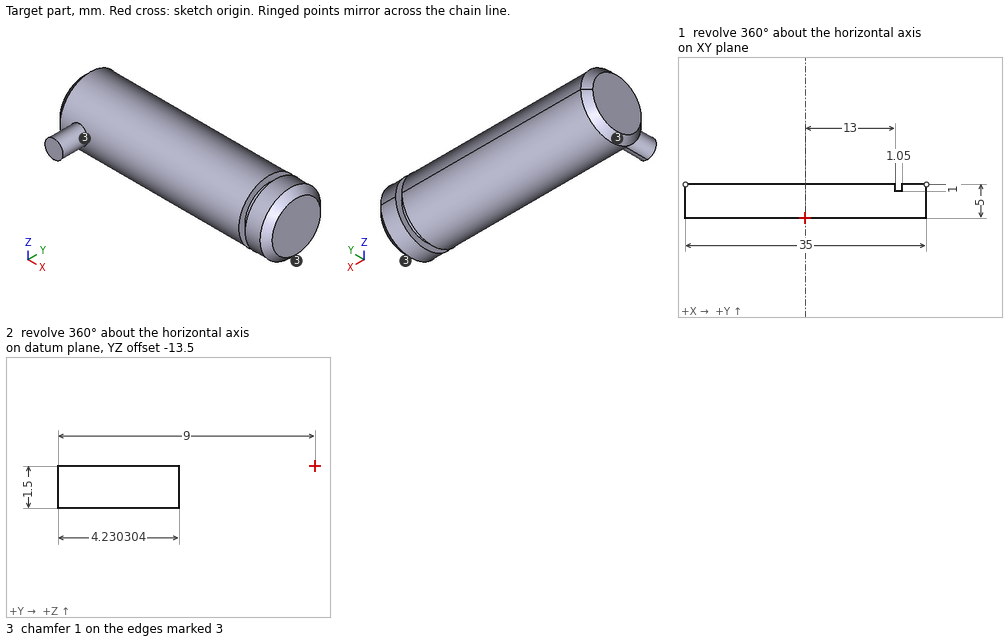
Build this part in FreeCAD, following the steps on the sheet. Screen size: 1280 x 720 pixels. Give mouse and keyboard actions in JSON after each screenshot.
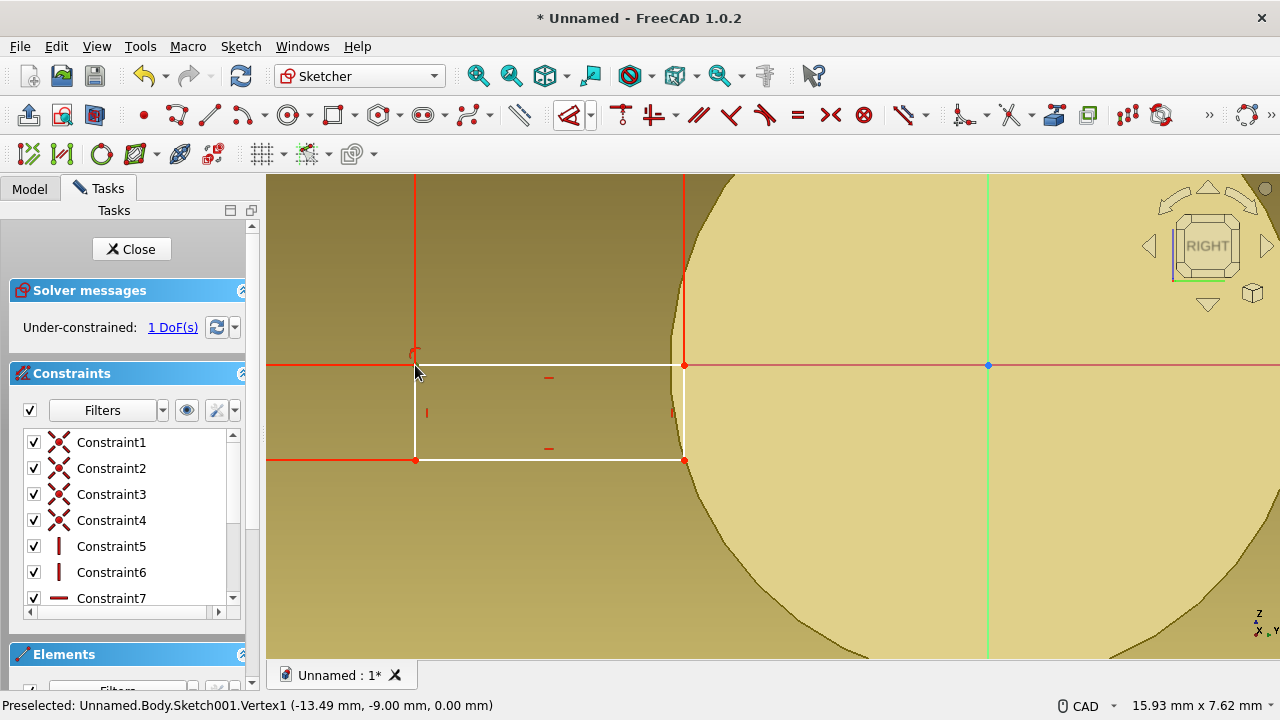
{"action": "key", "text": "l"}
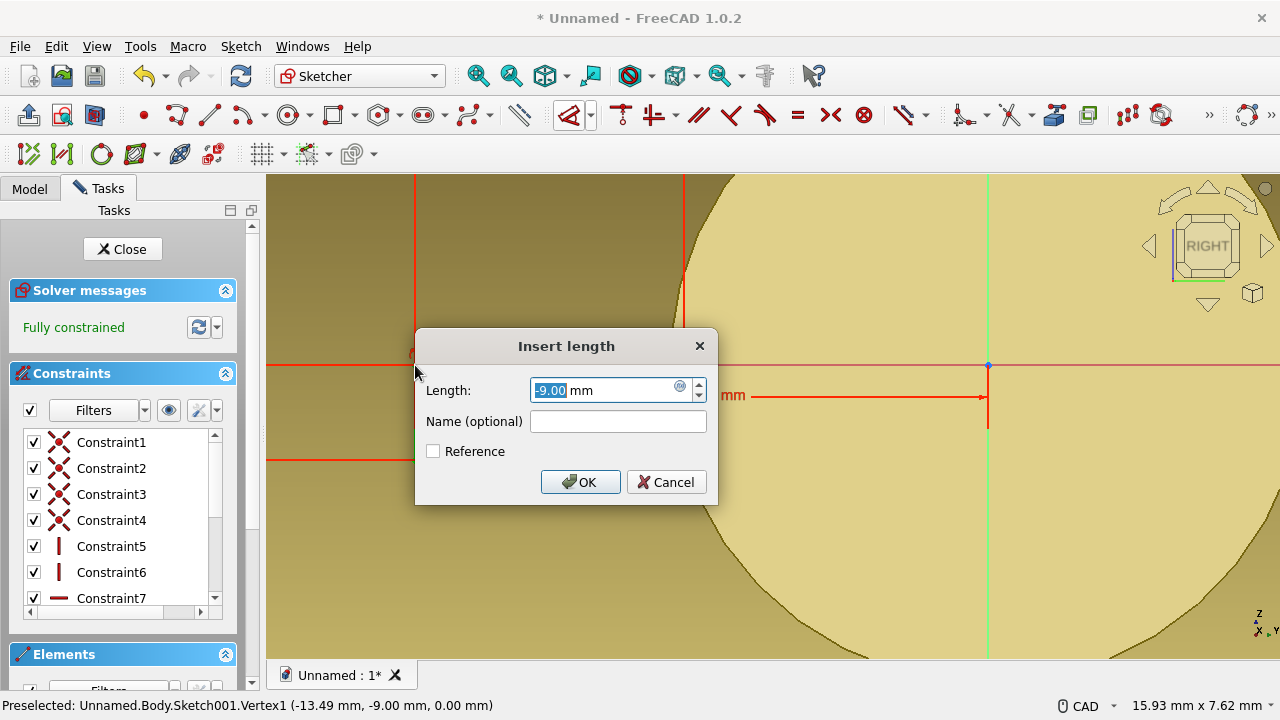
{"action": "type", "text": "-9"}
{"action": "key", "text": "Return"}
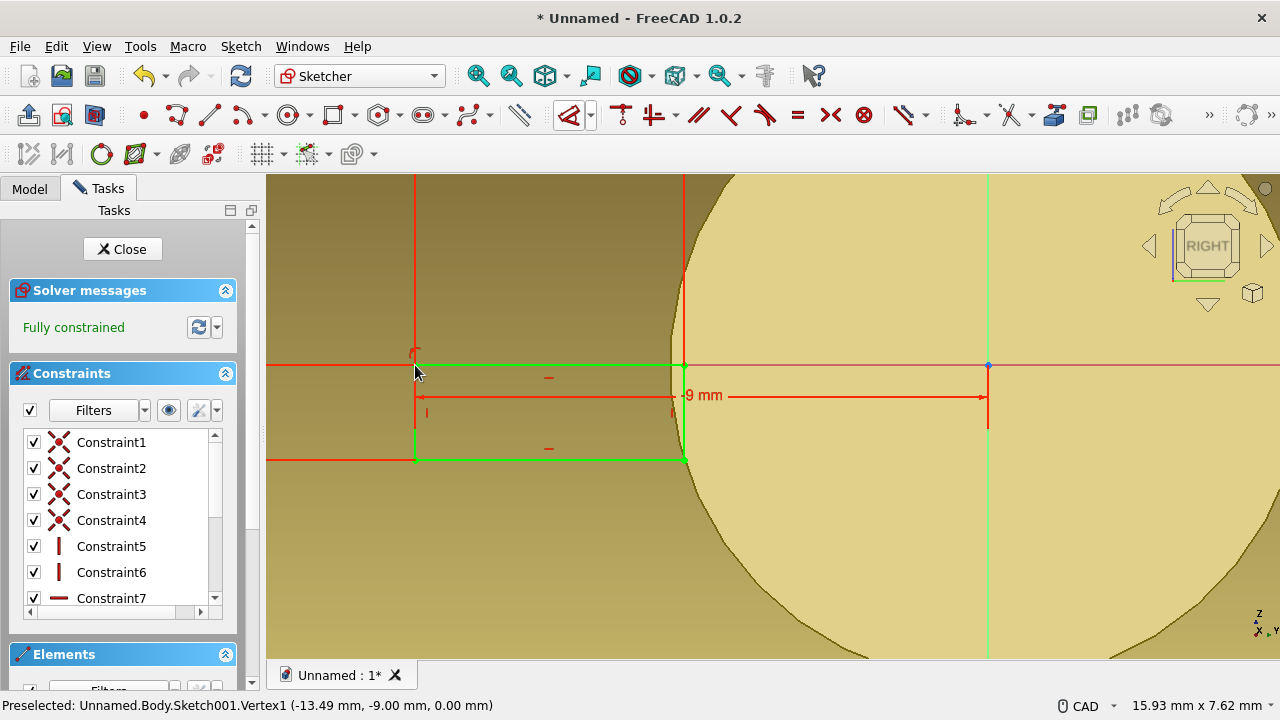
{"action": "left_click", "coordinate": [123, 249]}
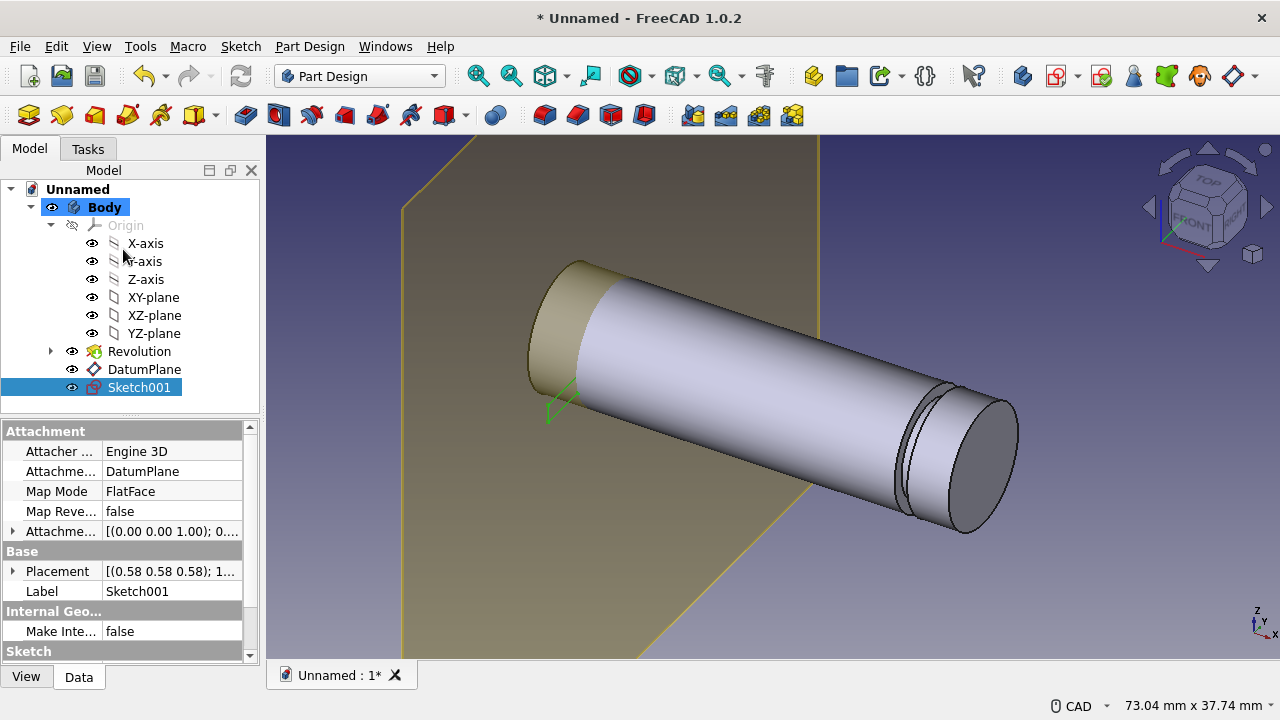
{"action": "left_click", "coordinate": [62, 116]}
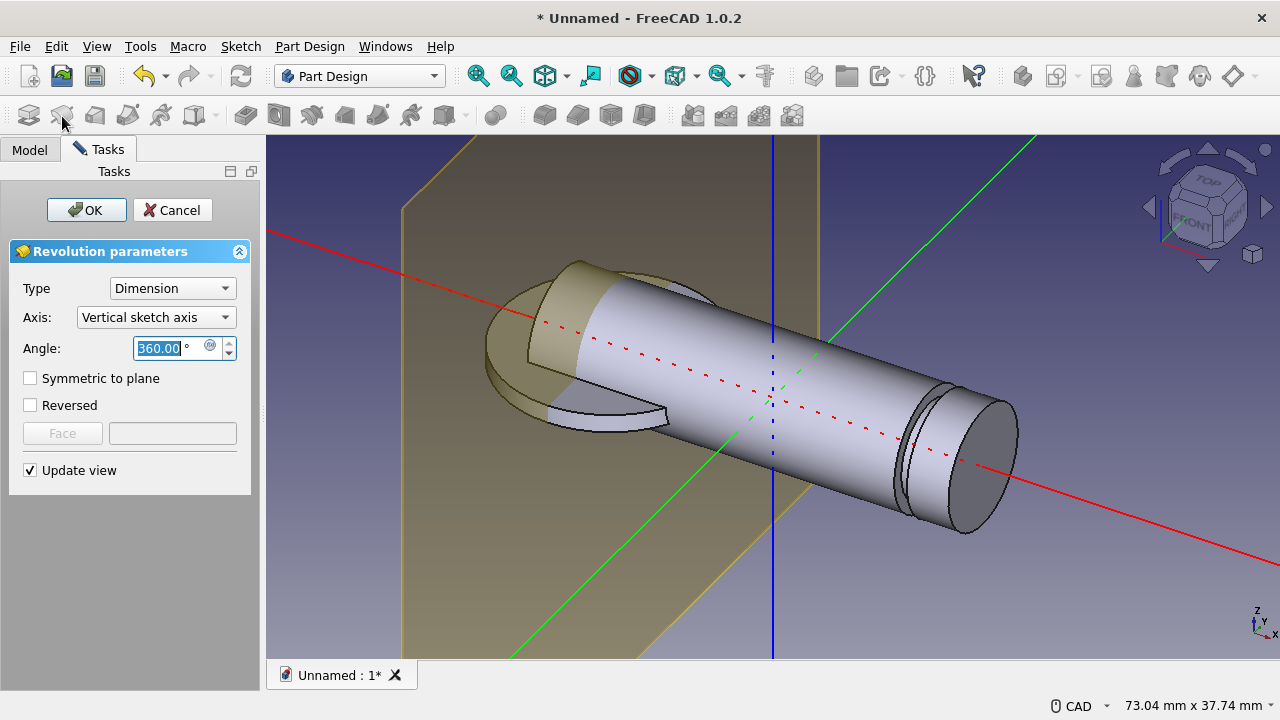
{"action": "left_click", "coordinate": [157, 318]}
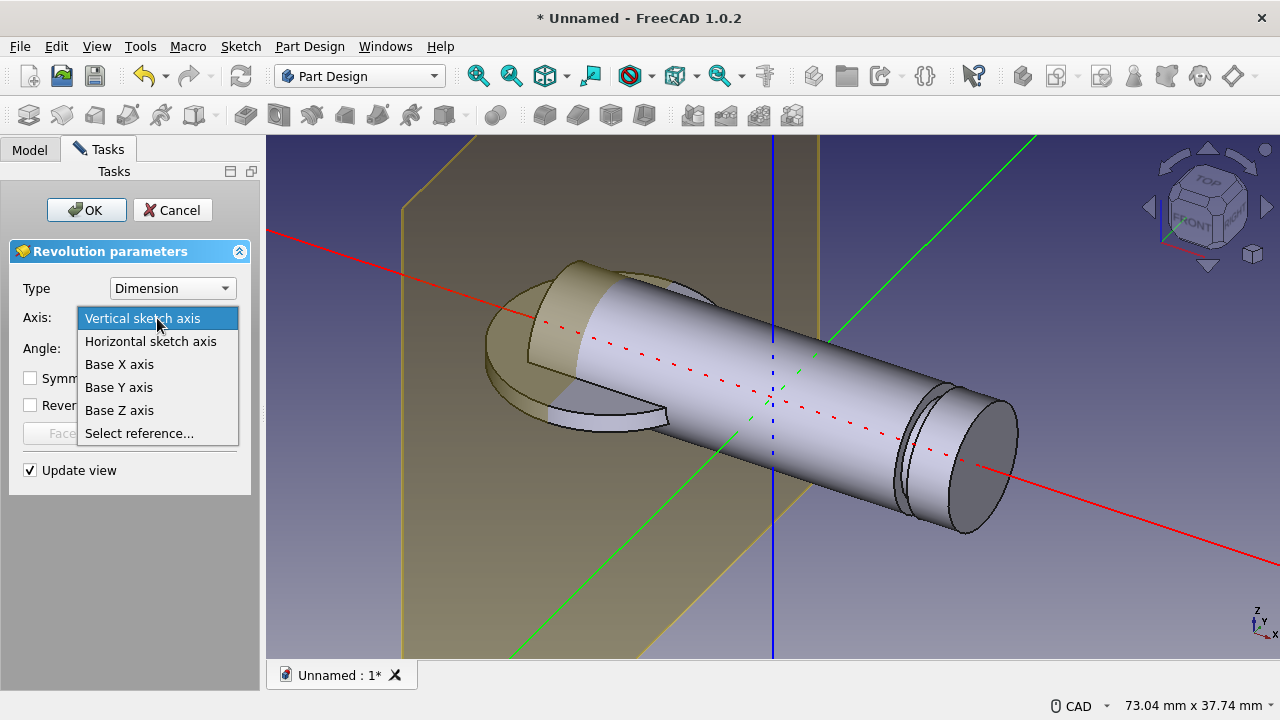
{"action": "left_click", "coordinate": [156, 342]}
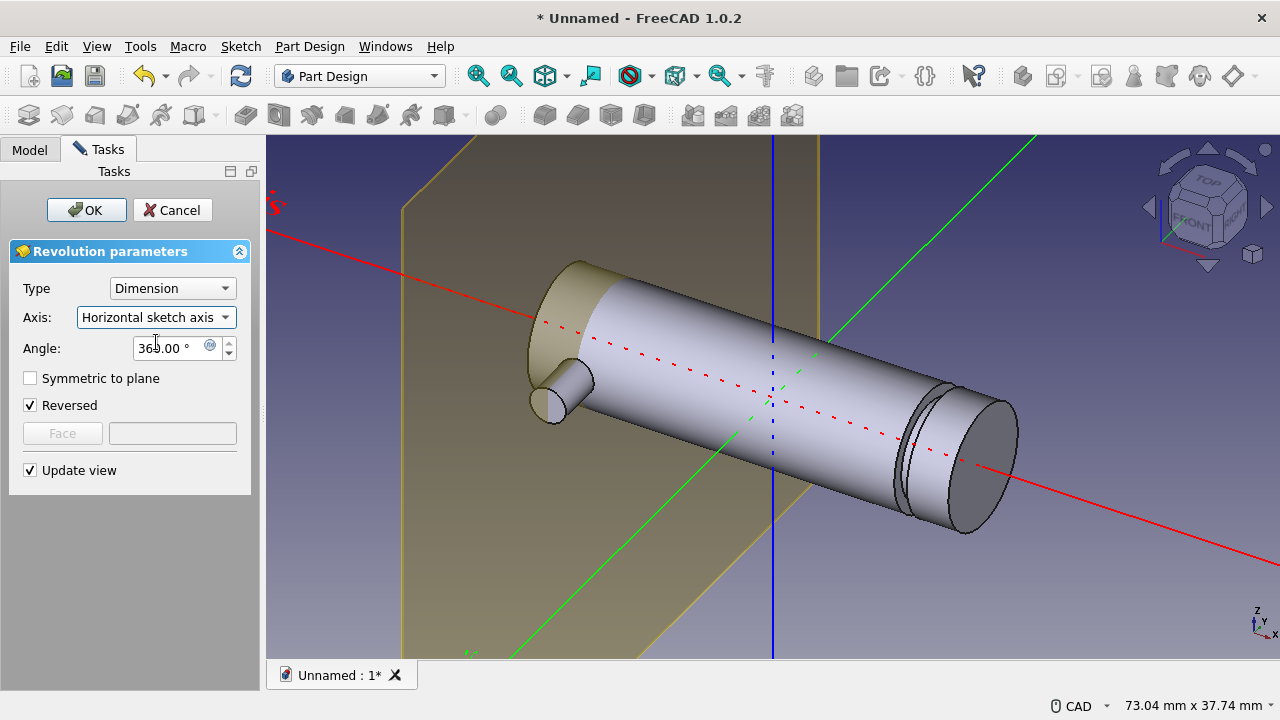
{"action": "left_click", "coordinate": [87, 210]}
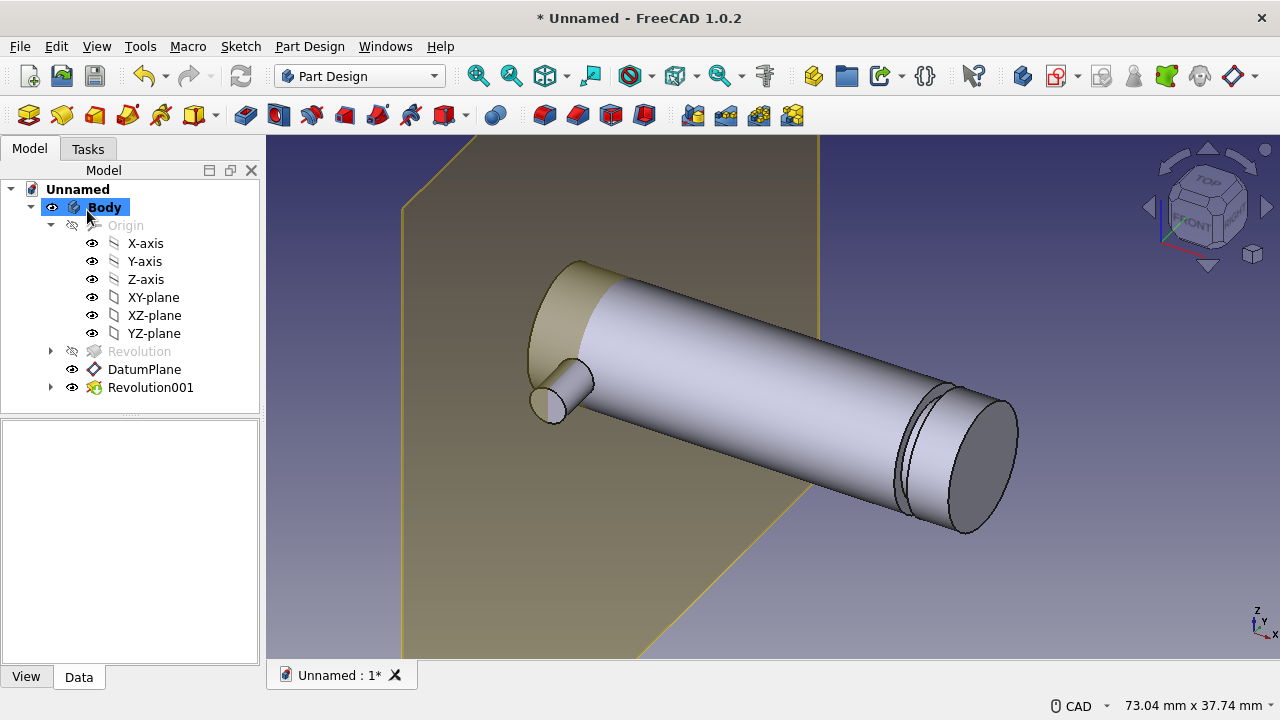
{"action": "left_click", "coordinate": [117, 369]}
{"action": "key", "text": "space"}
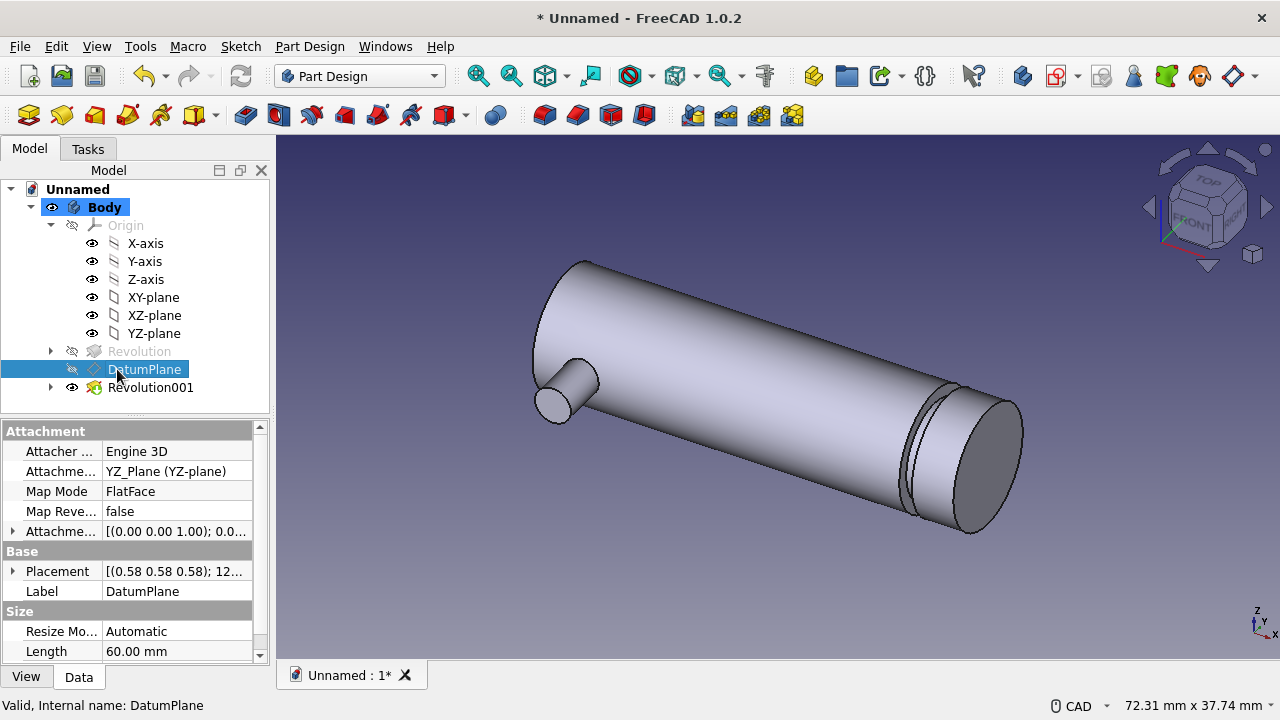
{"action": "left_click", "coordinate": [953, 500]}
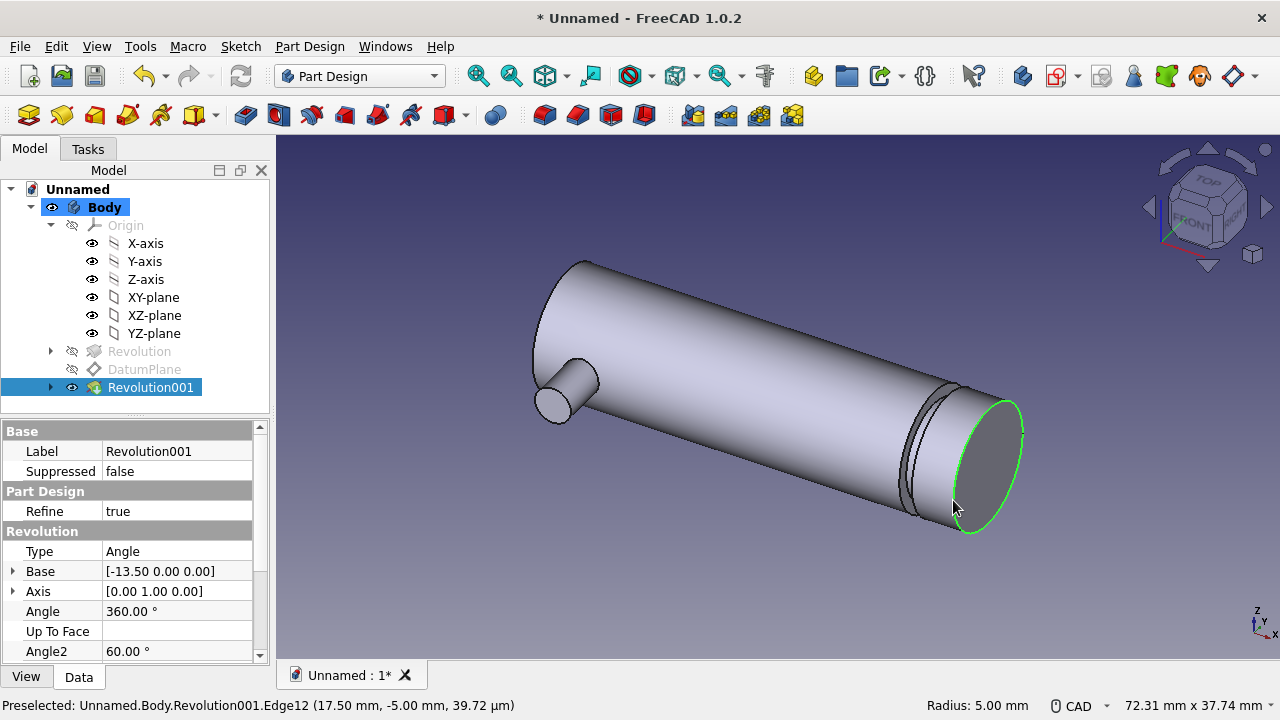
{"action": "key", "text": "0"}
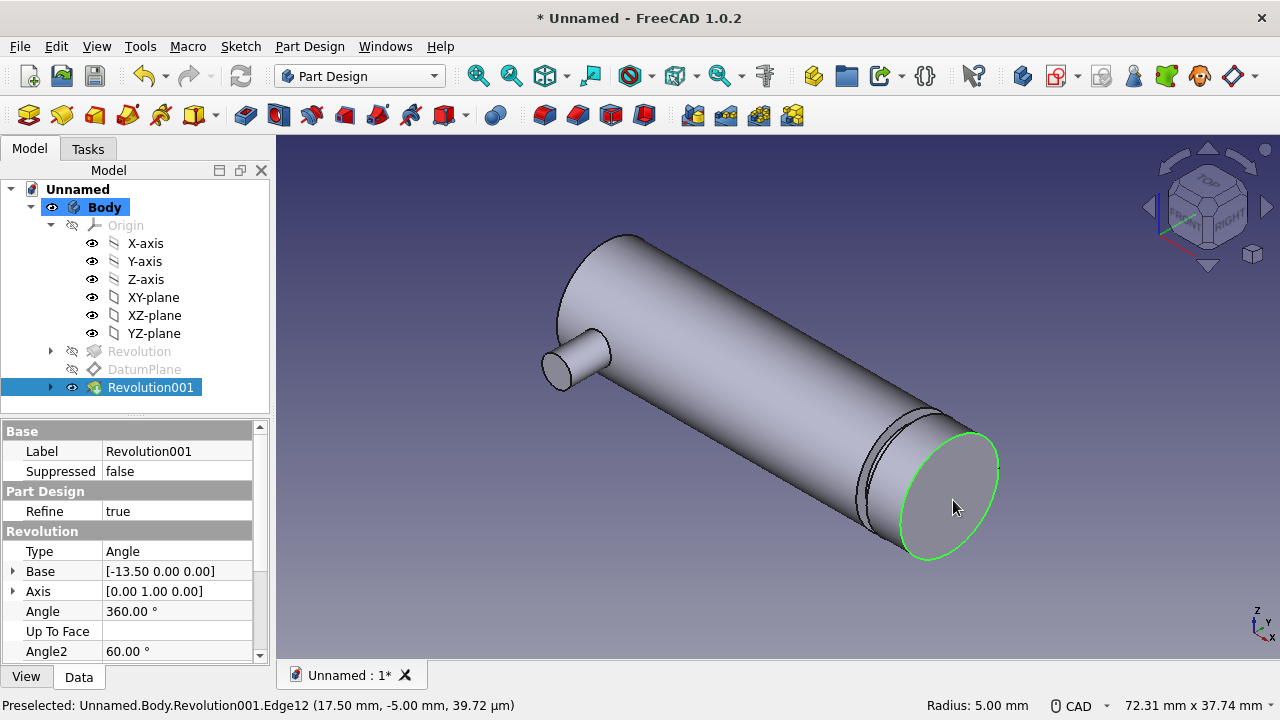
{"action": "key", "text": "2"}